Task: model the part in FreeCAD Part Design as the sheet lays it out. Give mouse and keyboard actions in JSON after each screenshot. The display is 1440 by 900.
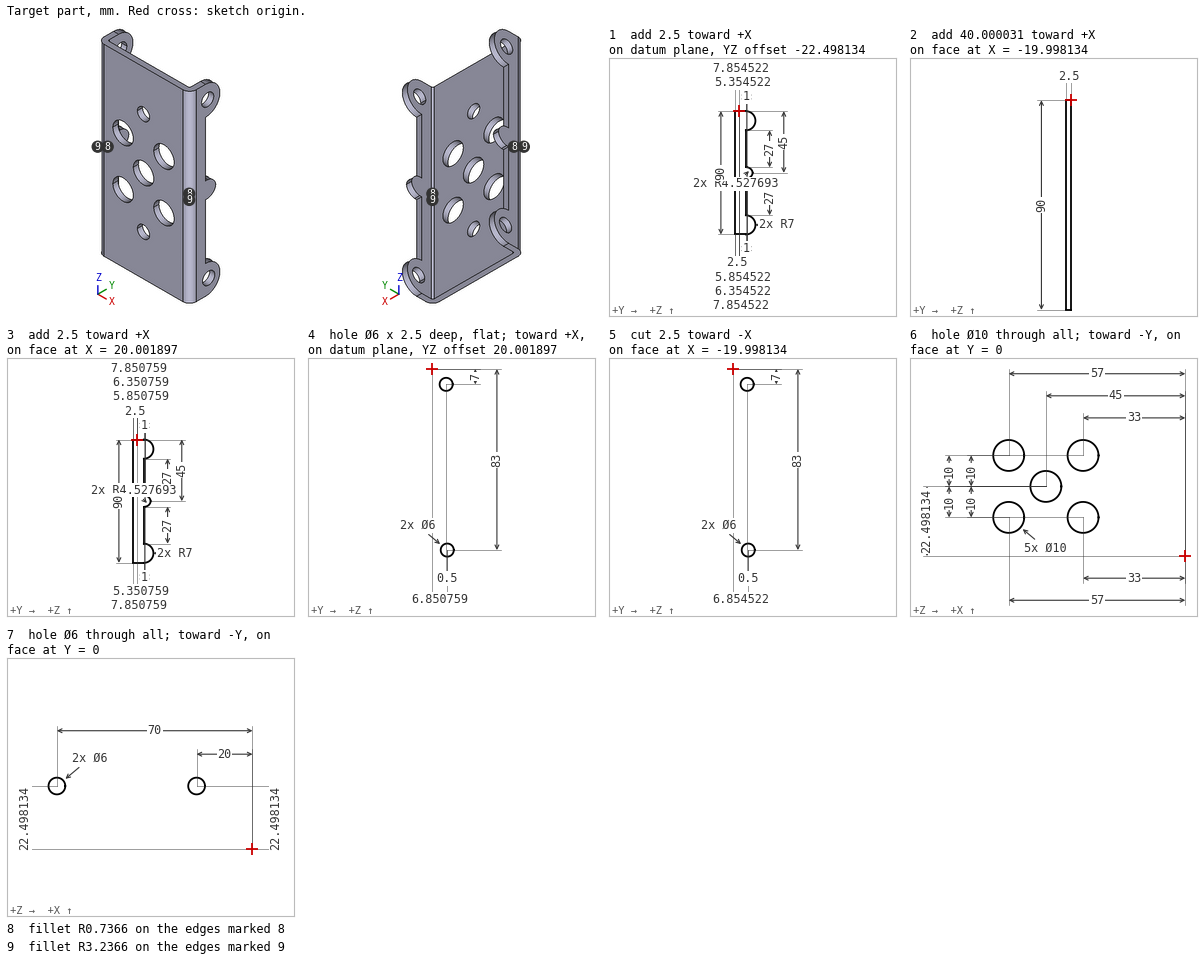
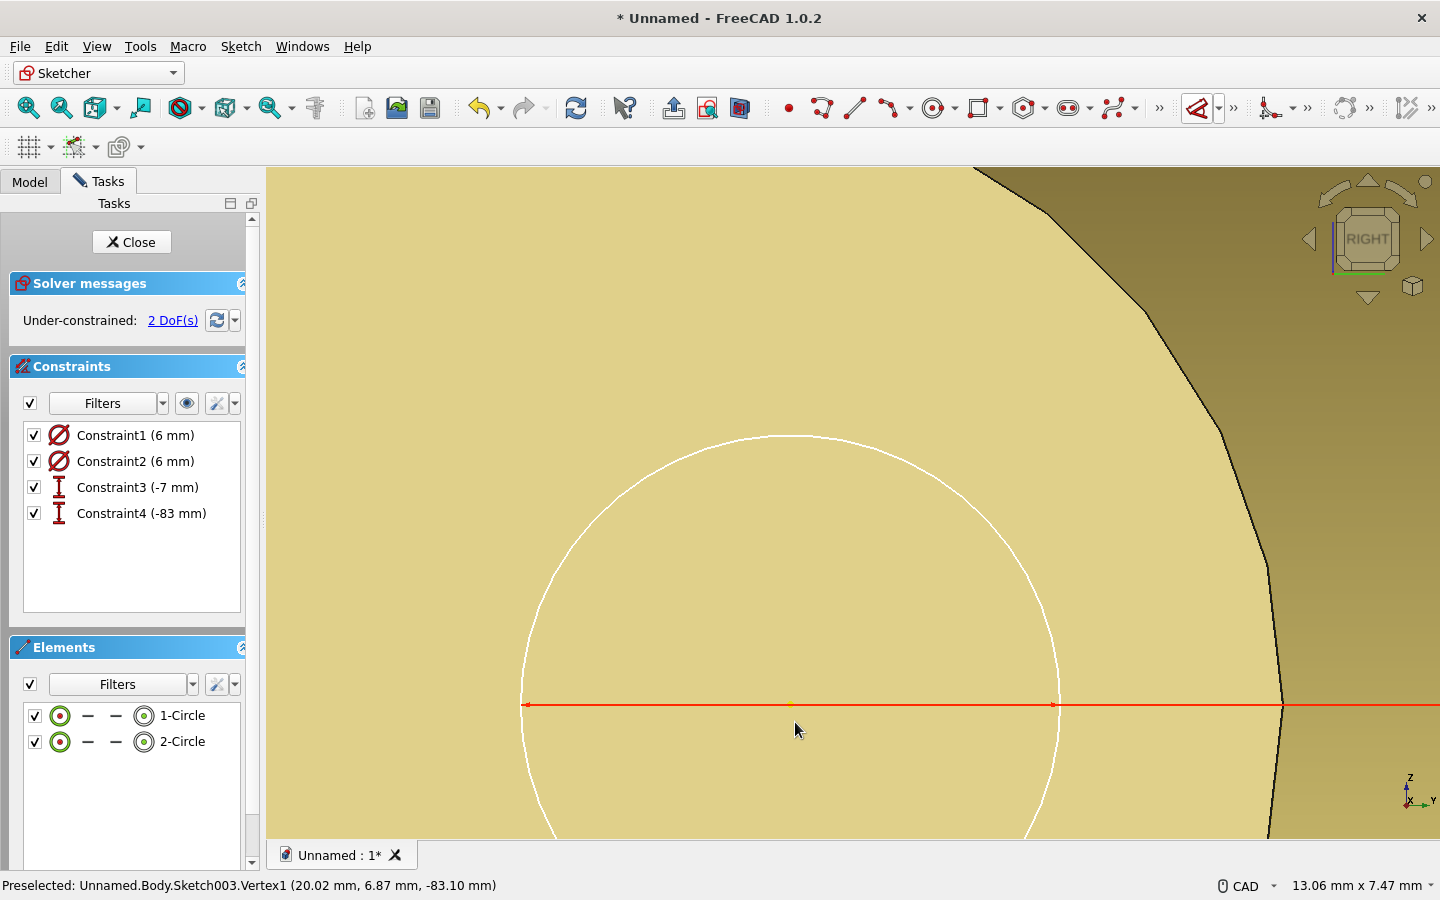
{"action": "left_click", "coordinate": [790, 705]}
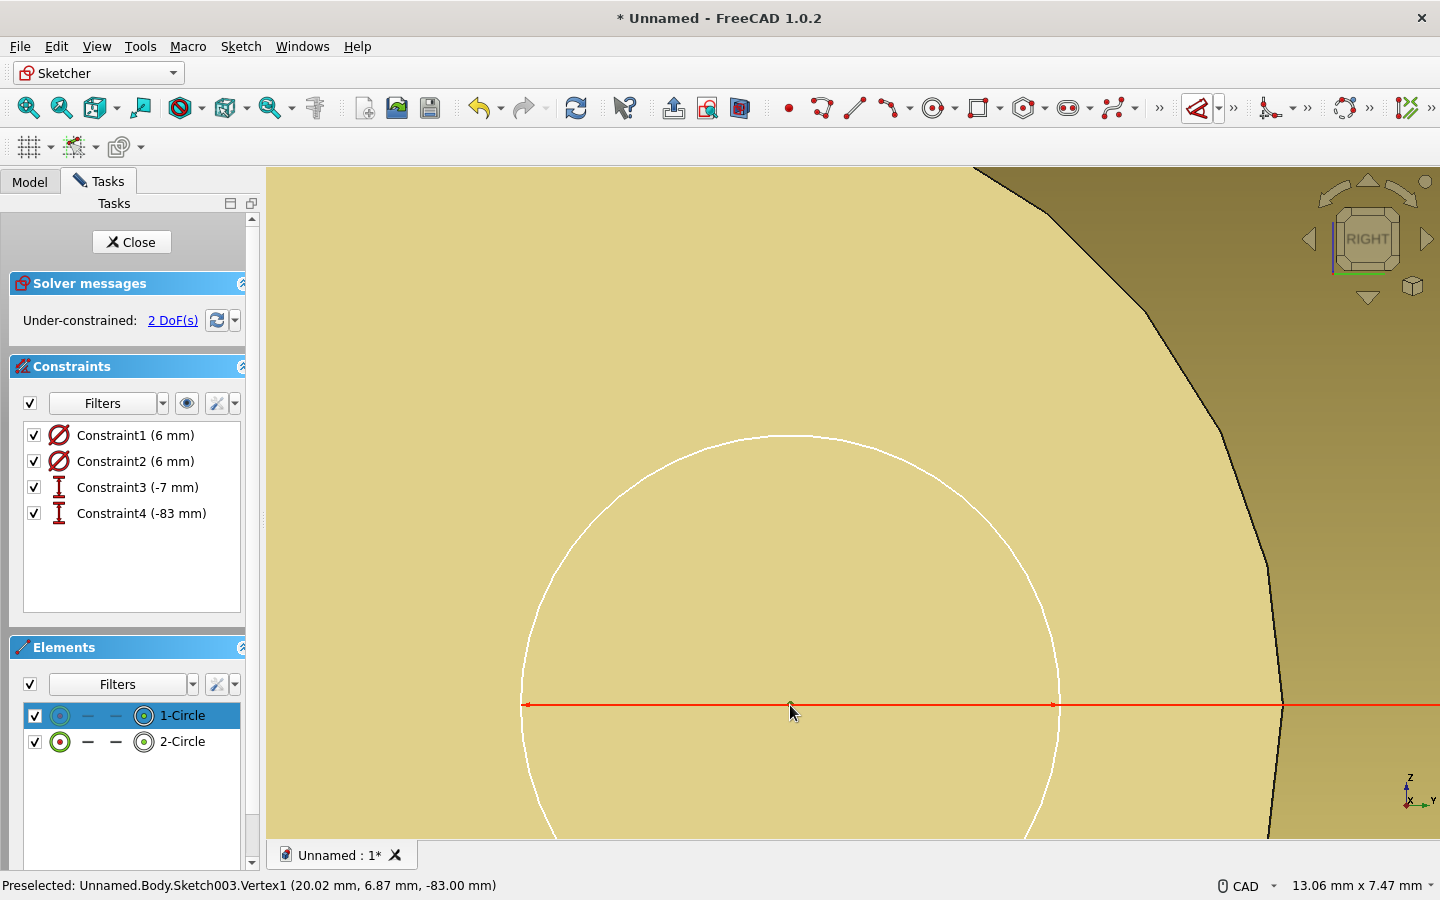
{"action": "scroll", "coordinate": [795, 723], "scroll_direction": "down", "scroll_amount": 14}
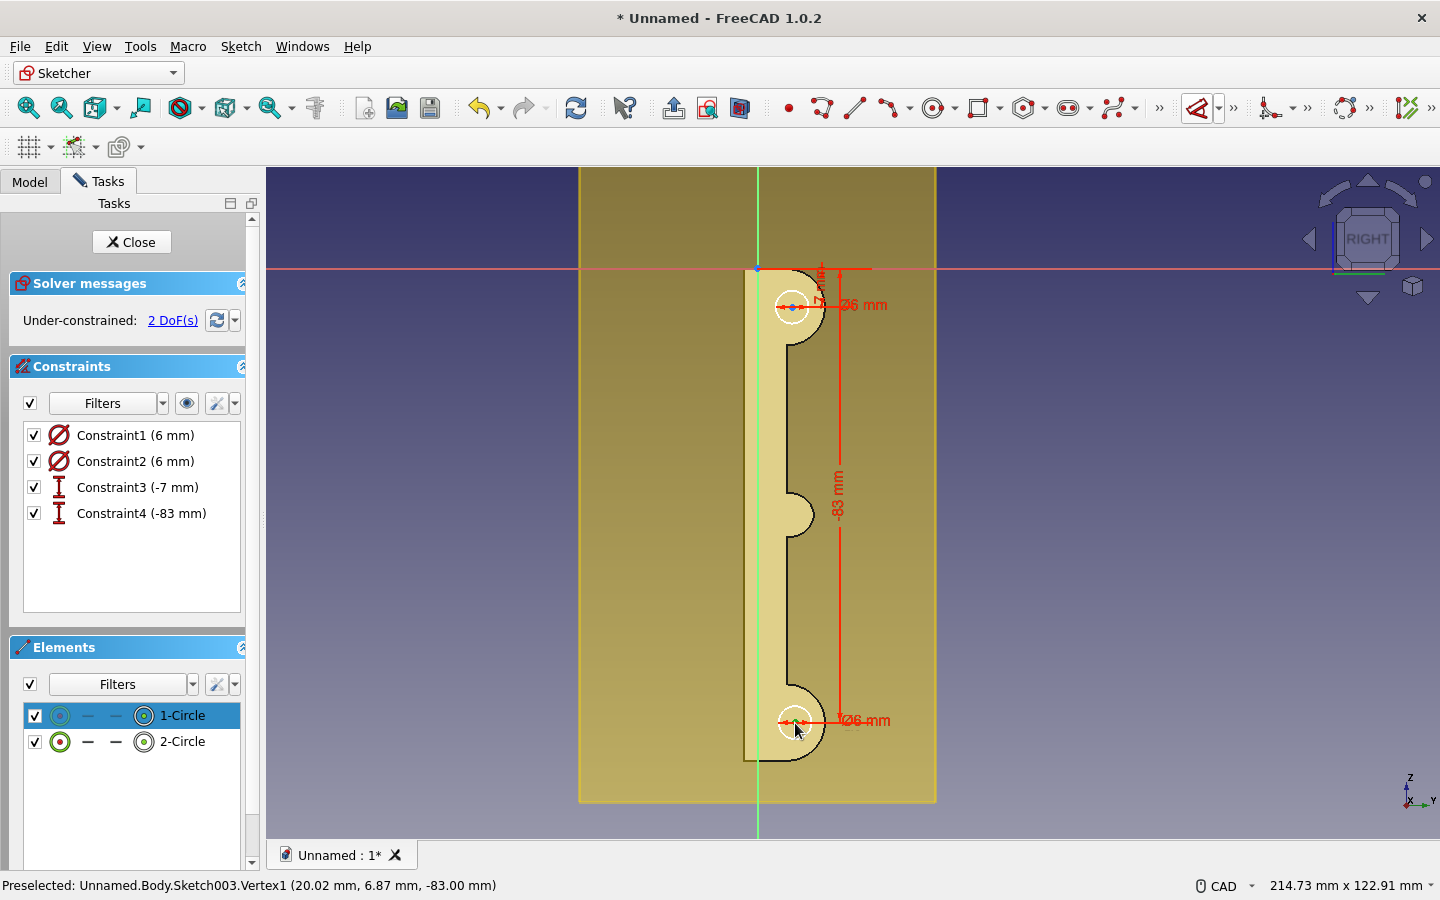
{"action": "scroll", "coordinate": [792, 307], "scroll_direction": "up", "scroll_amount": 14}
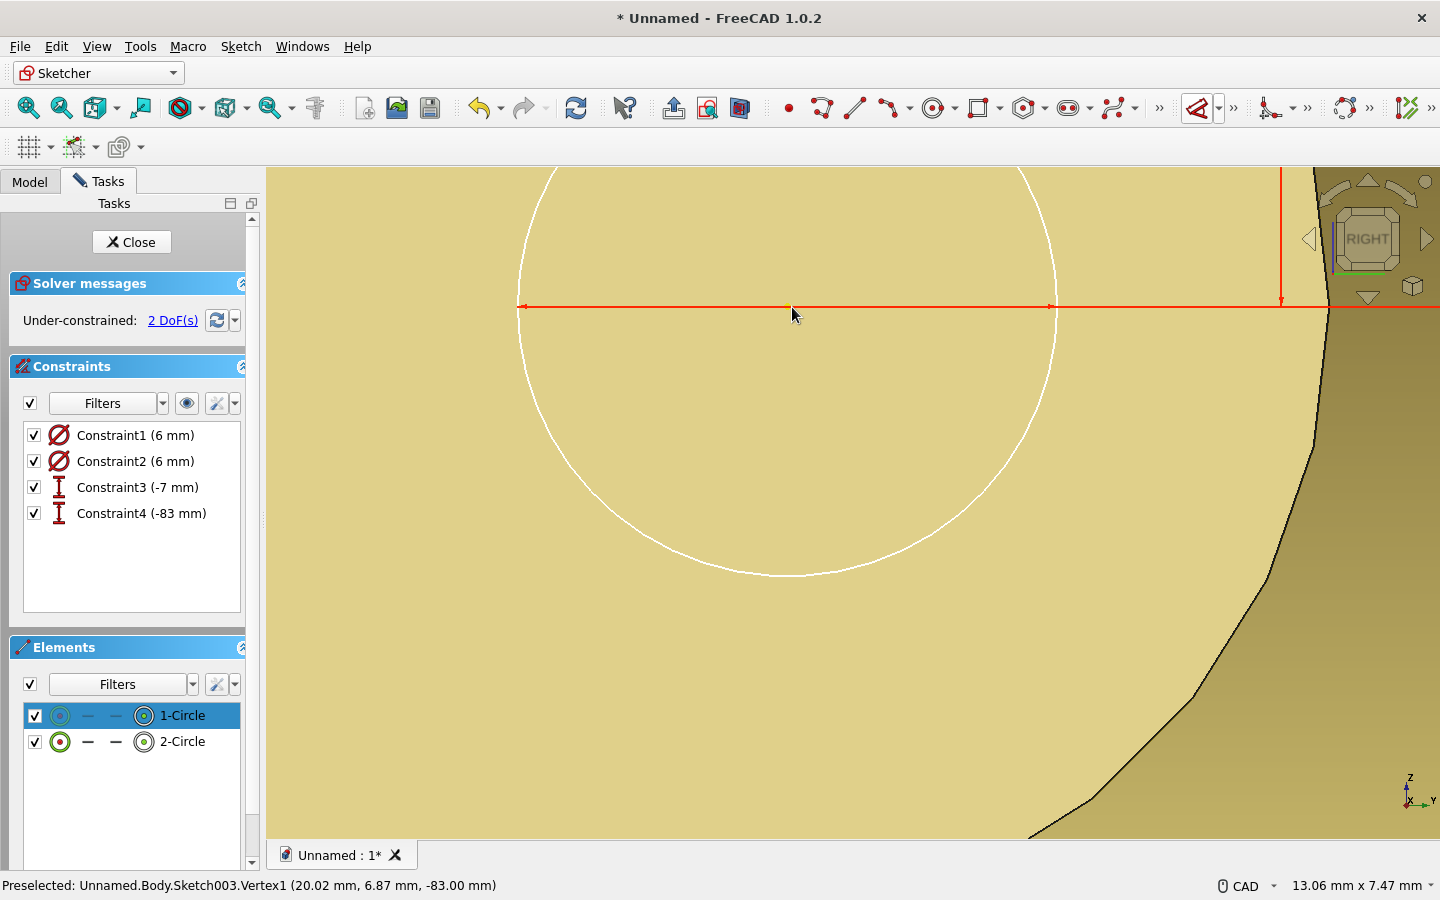
{"action": "left_click", "coordinate": [788, 307]}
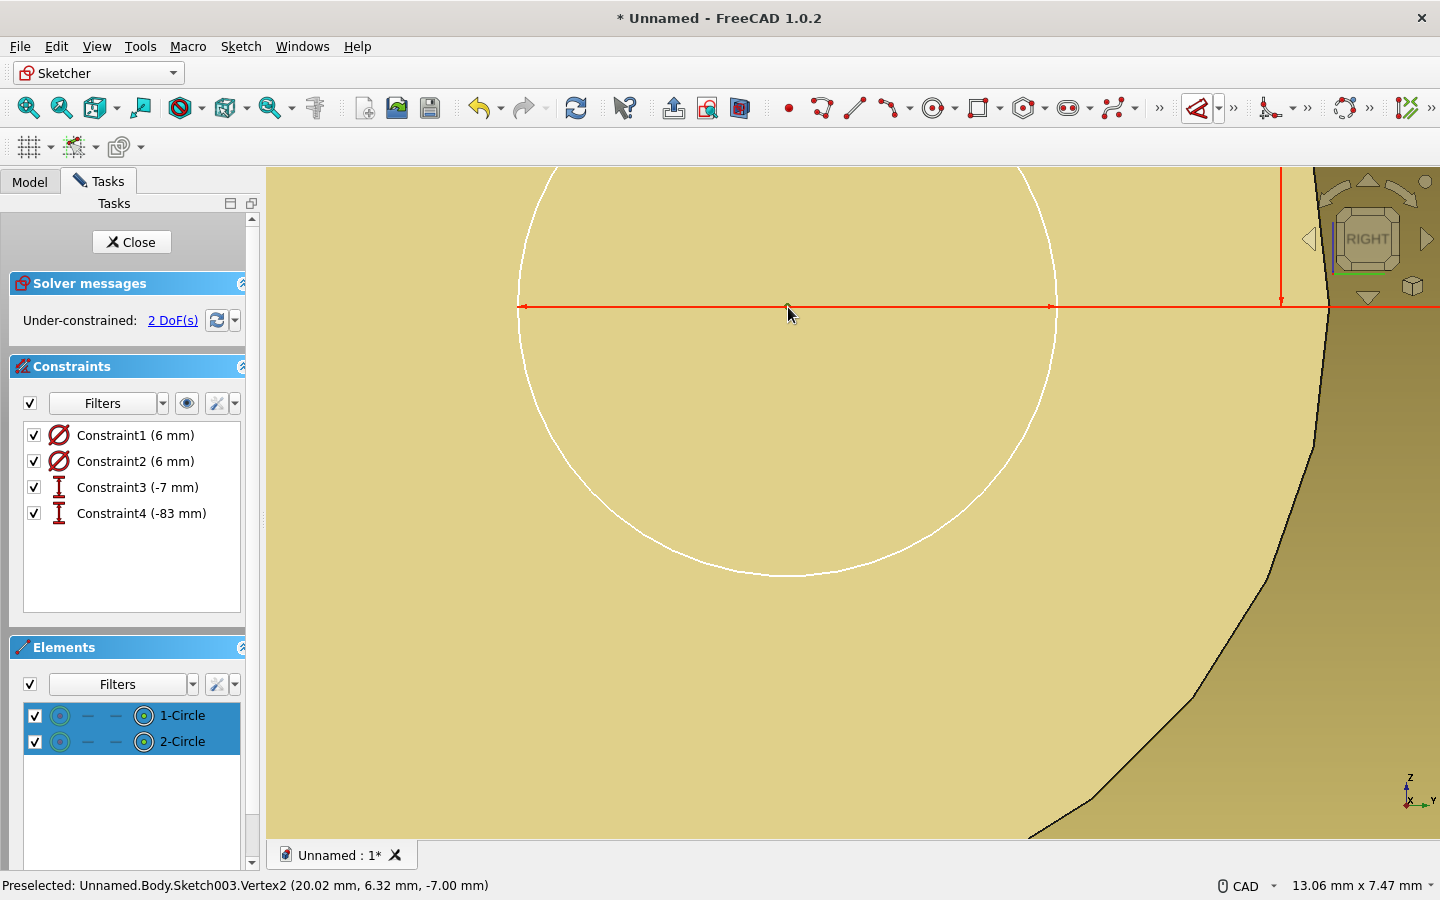
{"action": "key", "text": "l"}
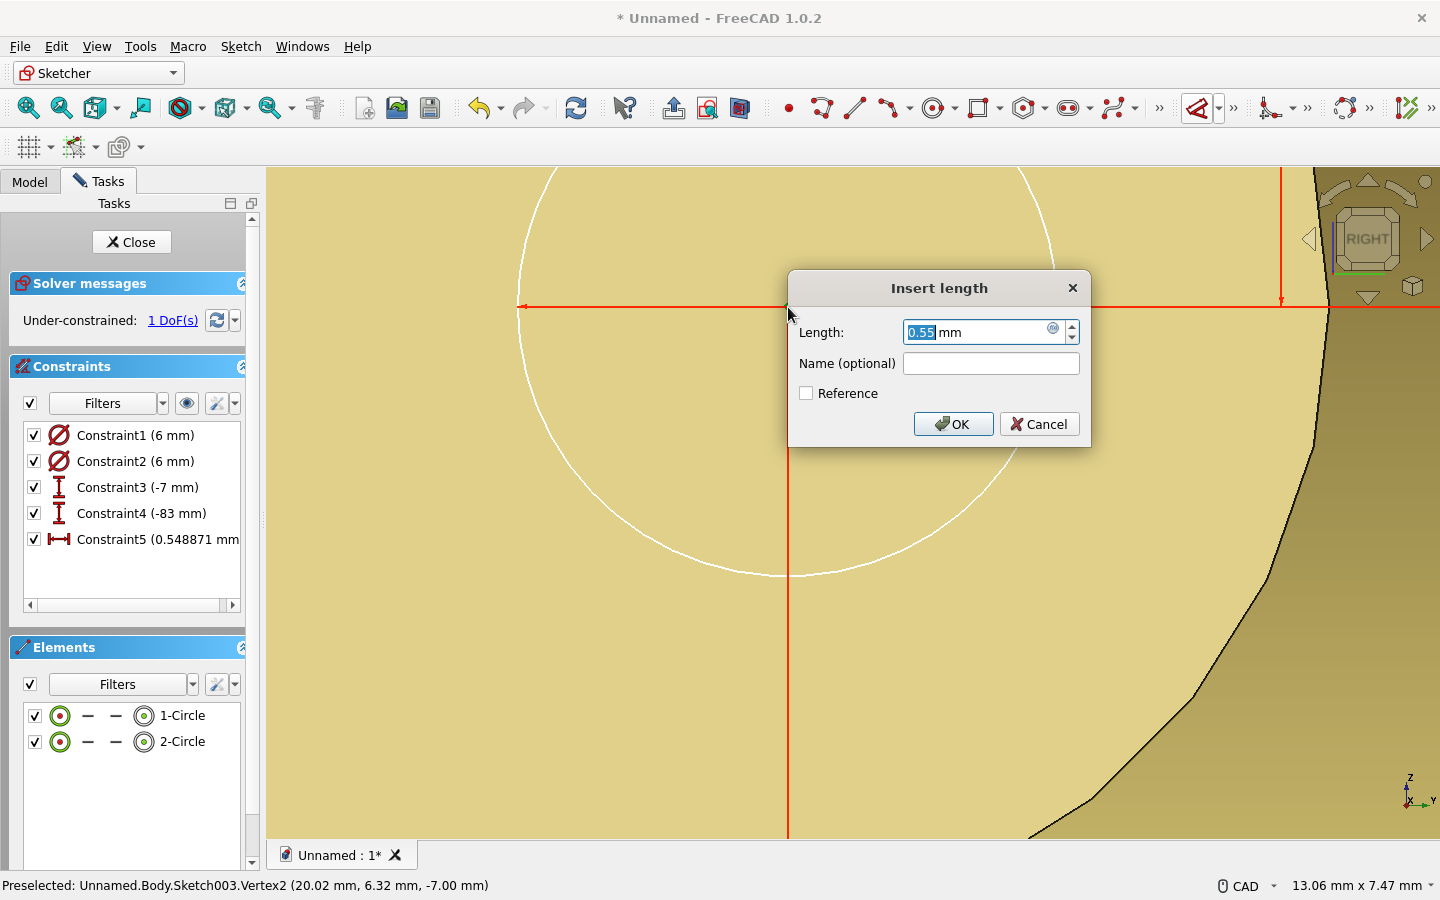
{"action": "type", "text": "0.5"}
{"action": "key", "text": "Return"}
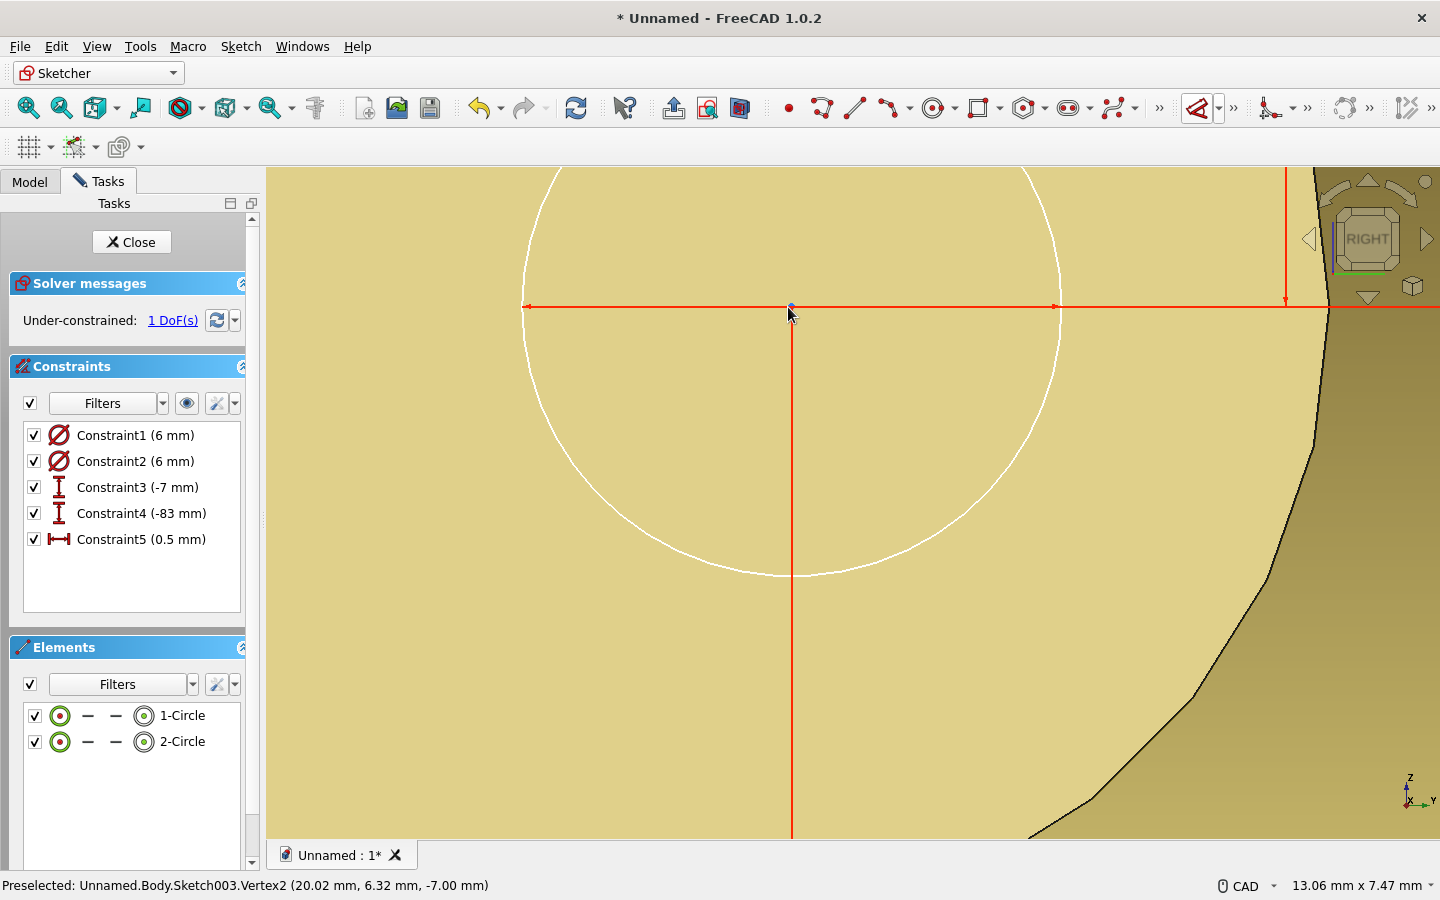
{"action": "scroll", "coordinate": [792, 306], "scroll_direction": "down", "scroll_amount": 14}